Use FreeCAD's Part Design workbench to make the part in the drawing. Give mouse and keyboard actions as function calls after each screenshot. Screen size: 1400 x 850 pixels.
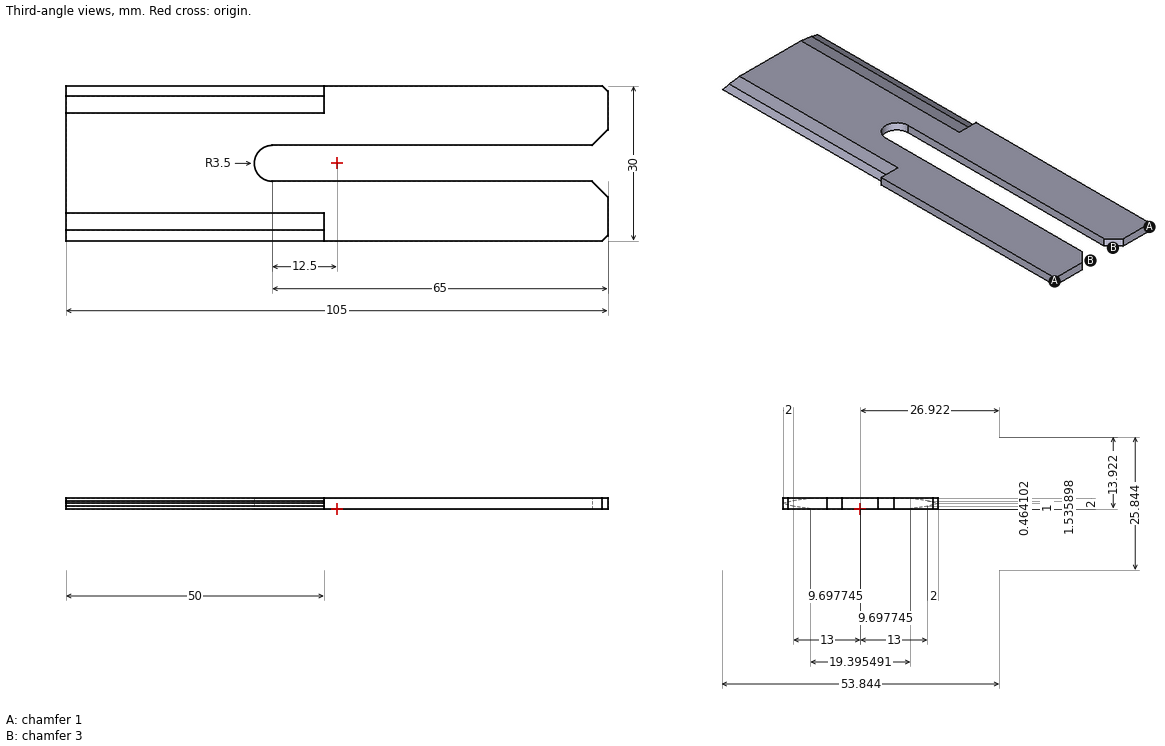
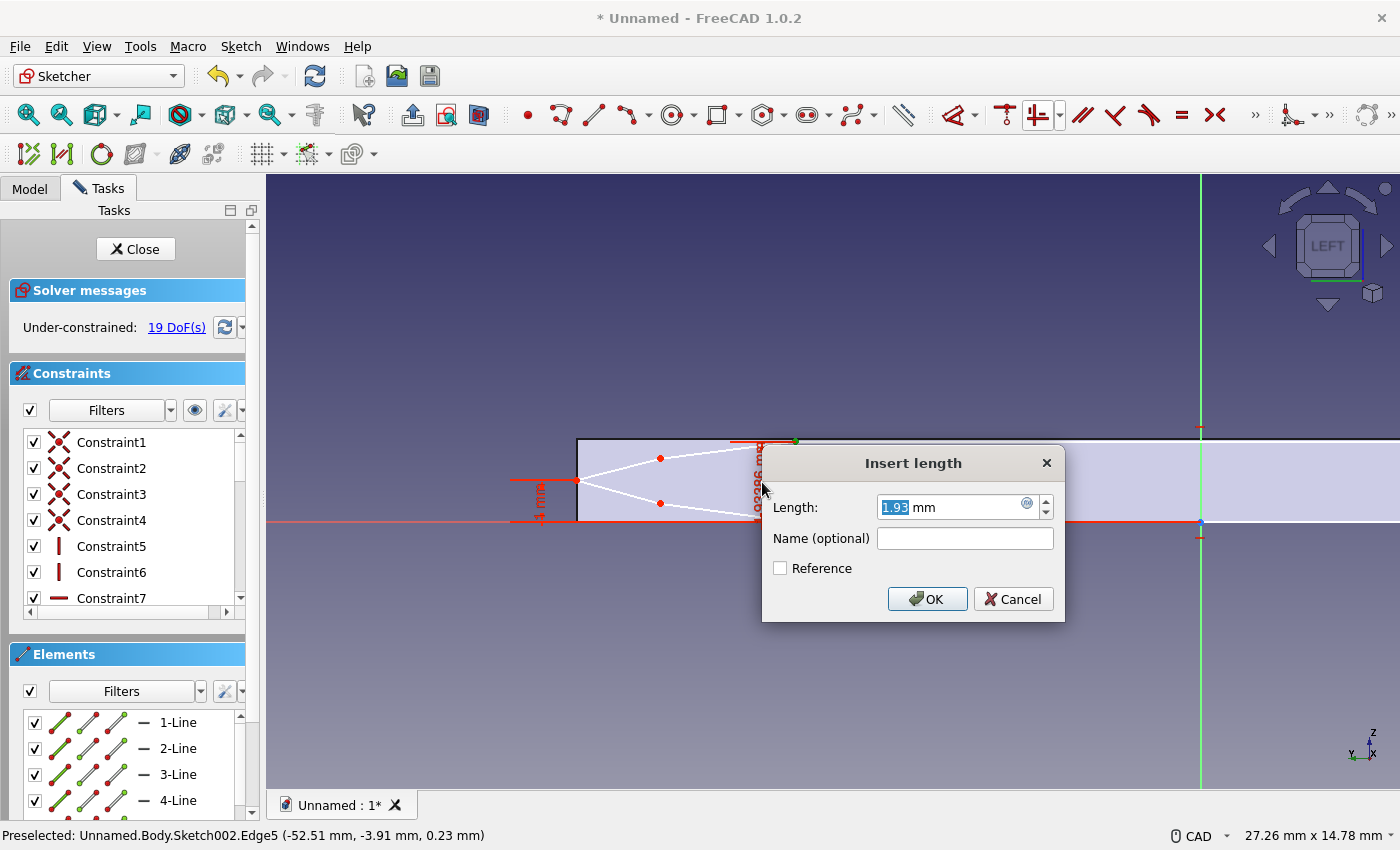
text(2)
key(Return)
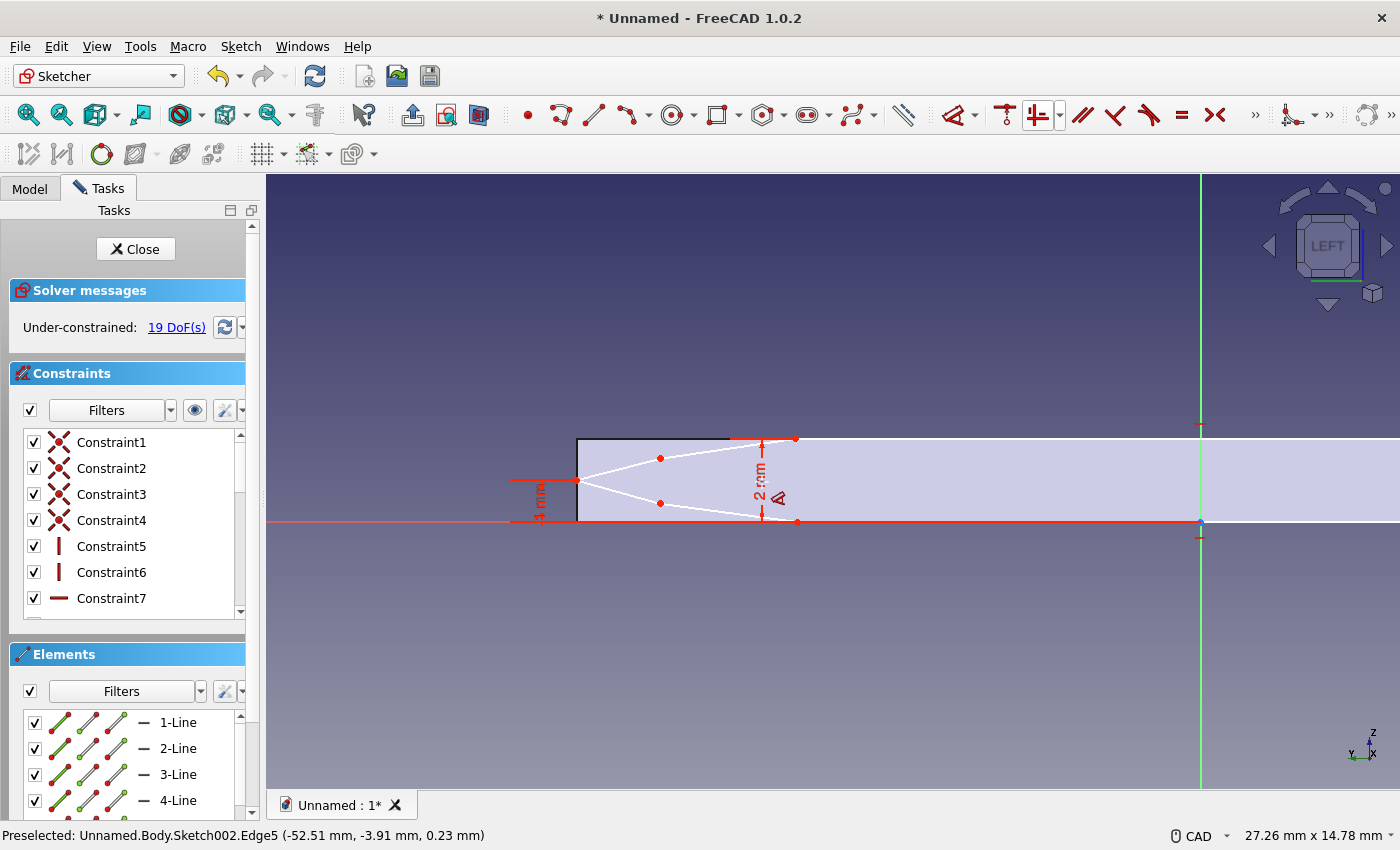
scroll(576, 482, down, 6)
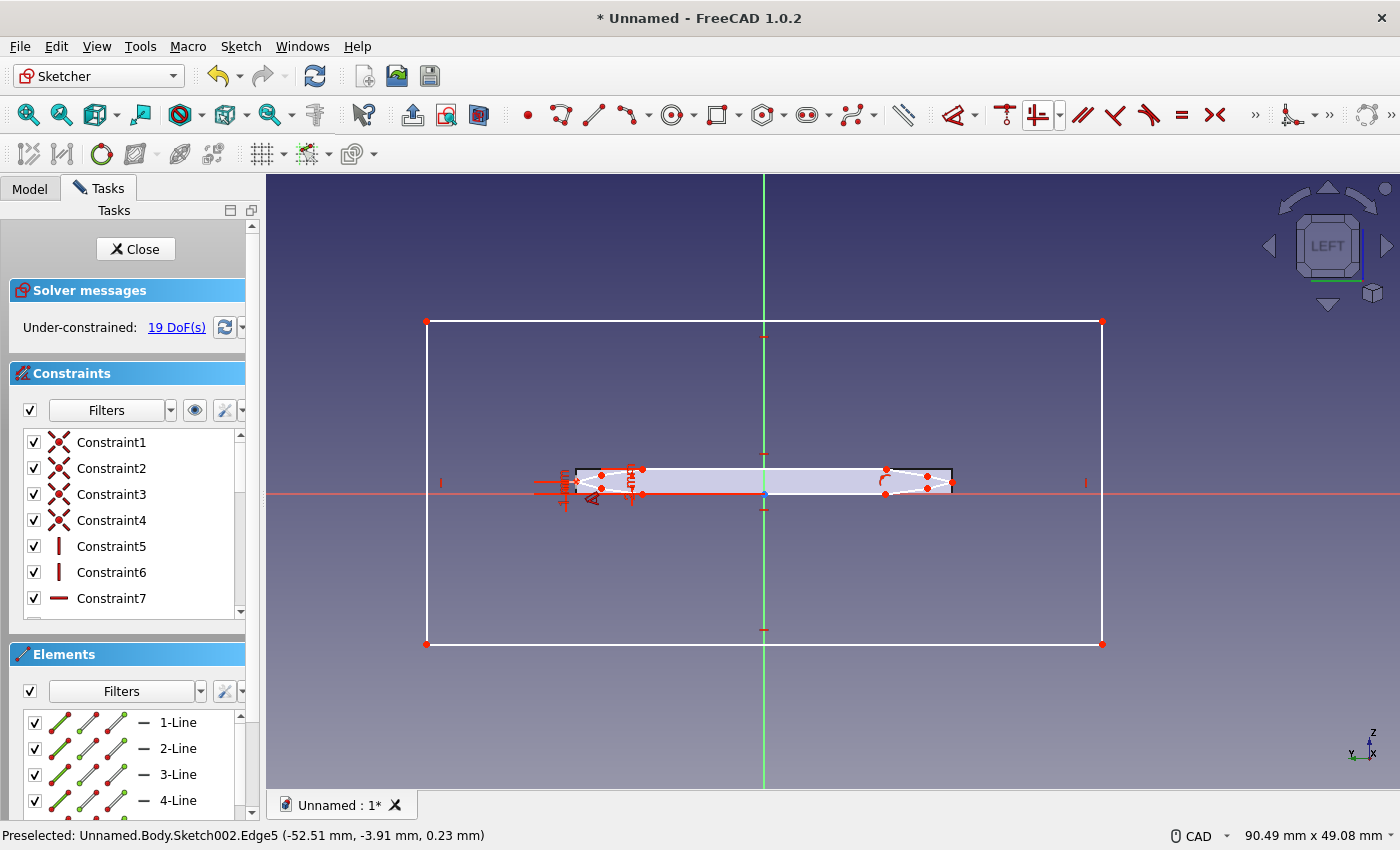
scroll(953, 482, up, 6)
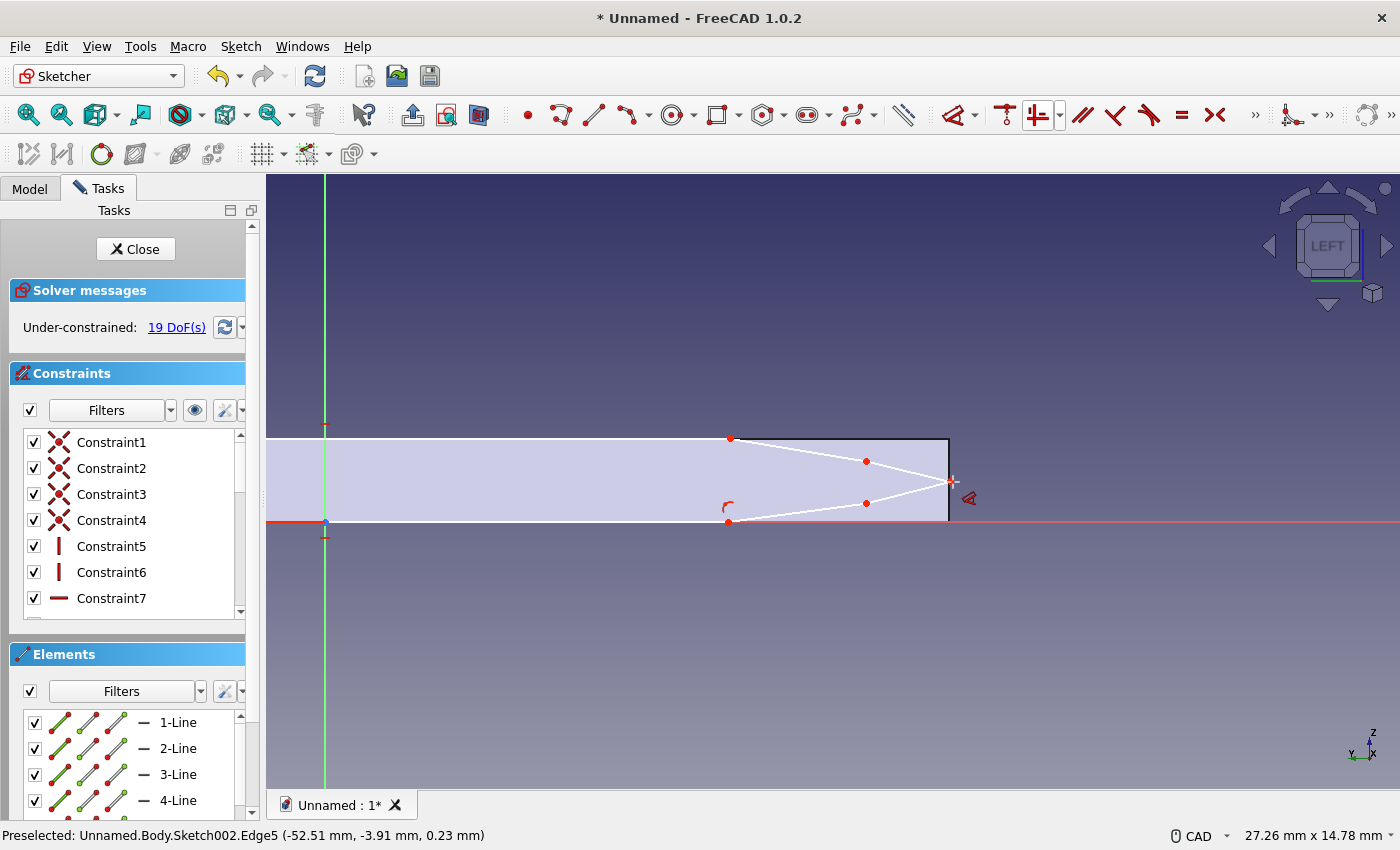
click(950, 482)
click(984, 502)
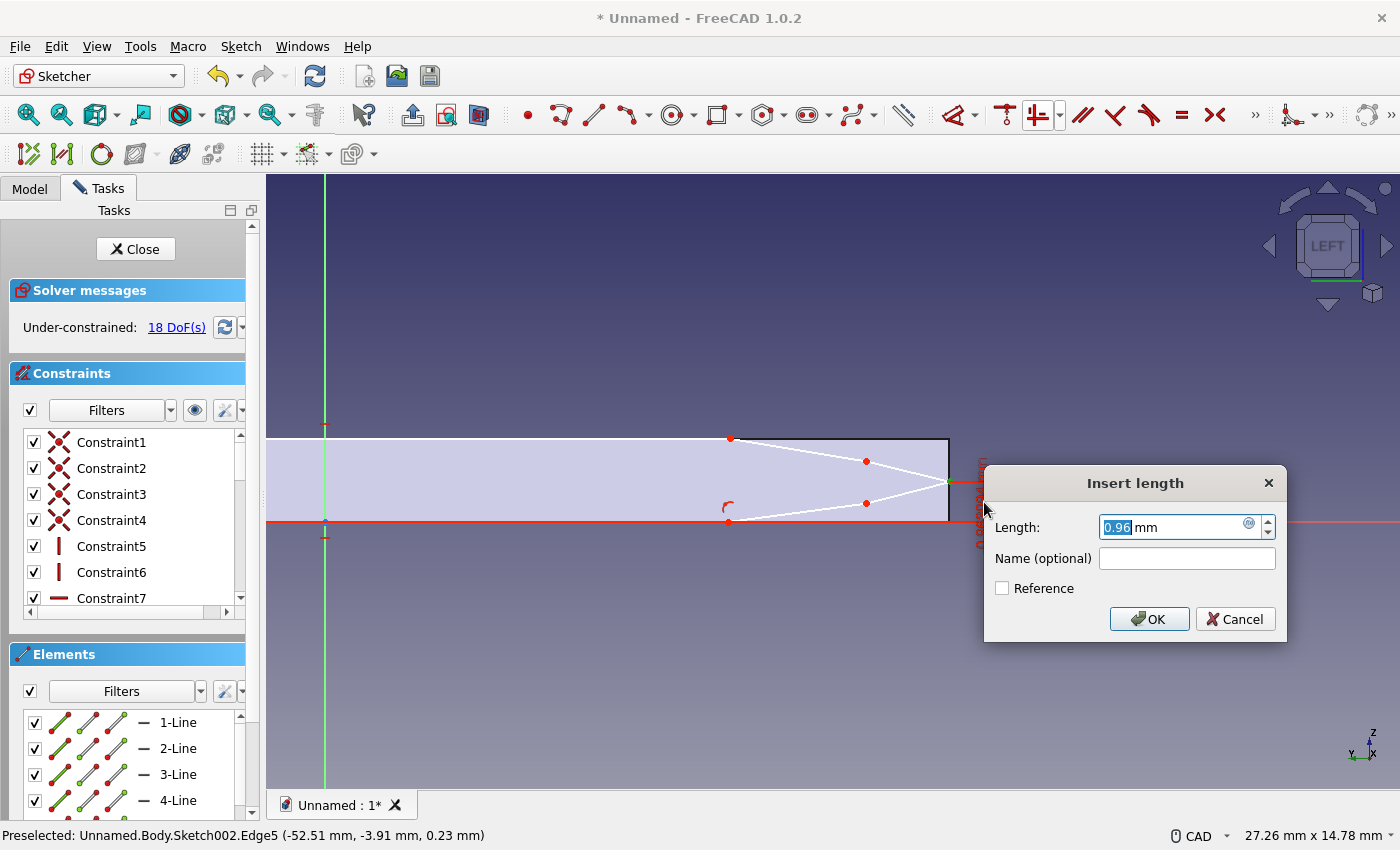
text(1)
key(Return)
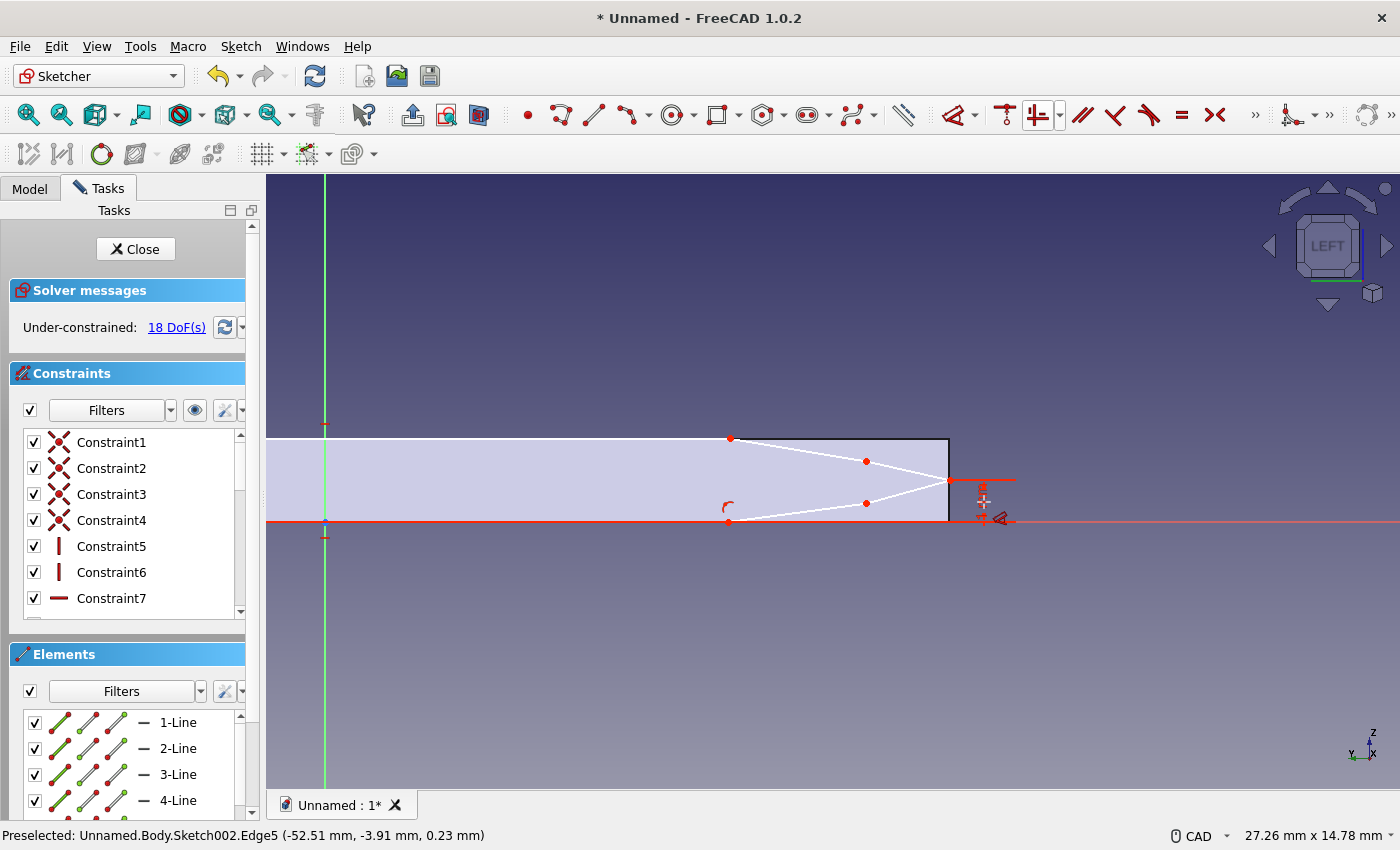
scroll(954, 482, down, 6)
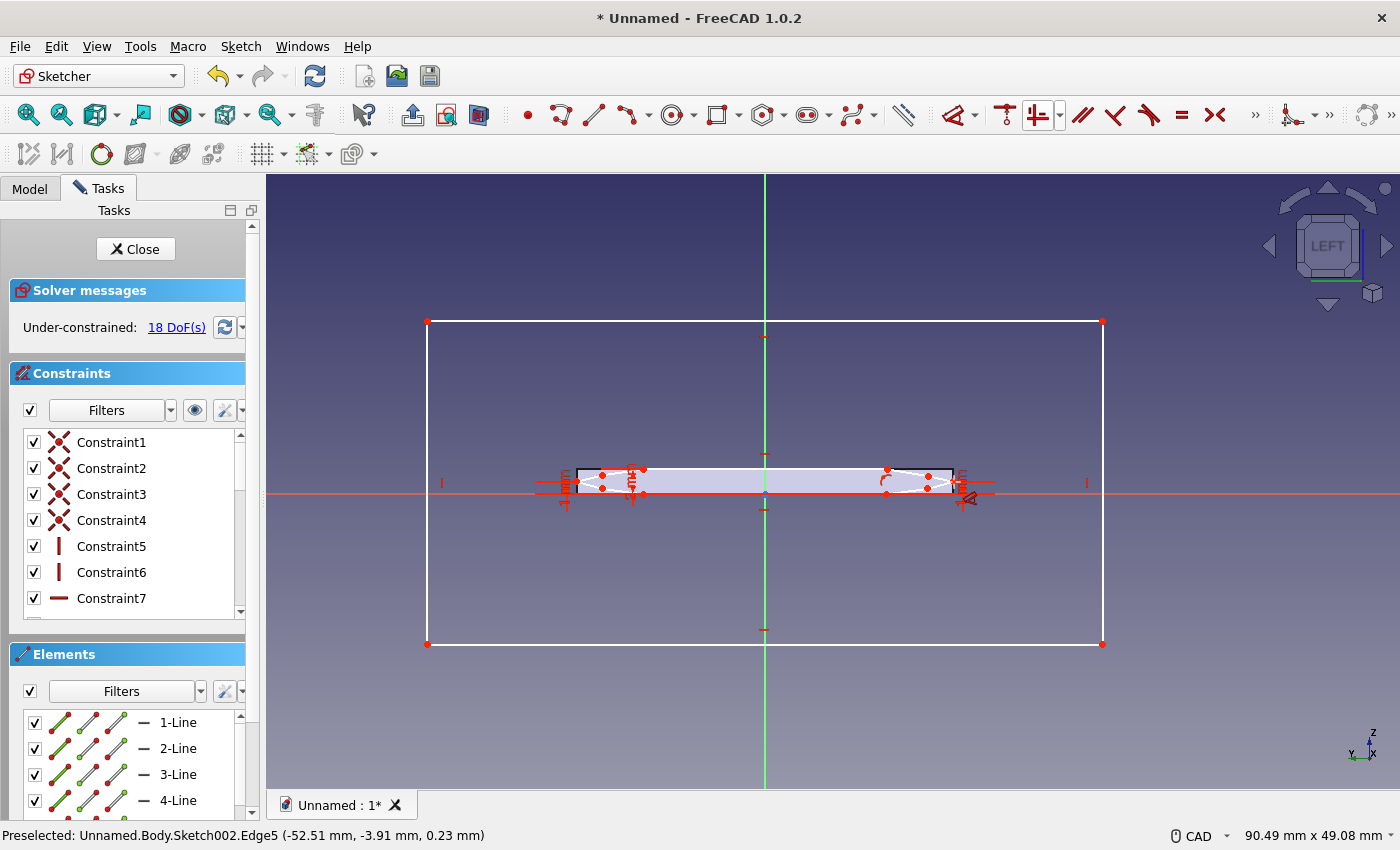
scroll(595, 487, up, 3)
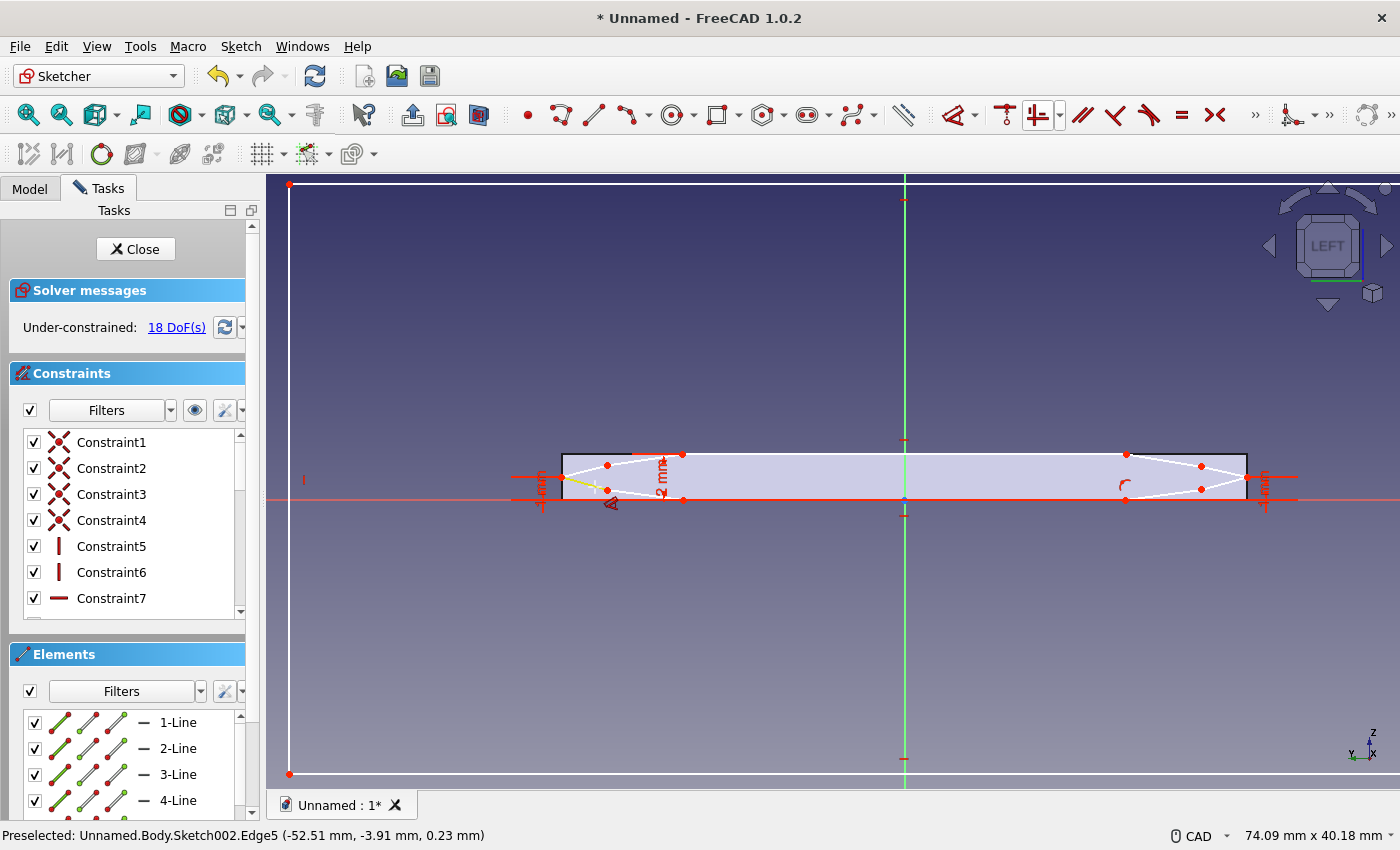
click(594, 486)
click(585, 524)